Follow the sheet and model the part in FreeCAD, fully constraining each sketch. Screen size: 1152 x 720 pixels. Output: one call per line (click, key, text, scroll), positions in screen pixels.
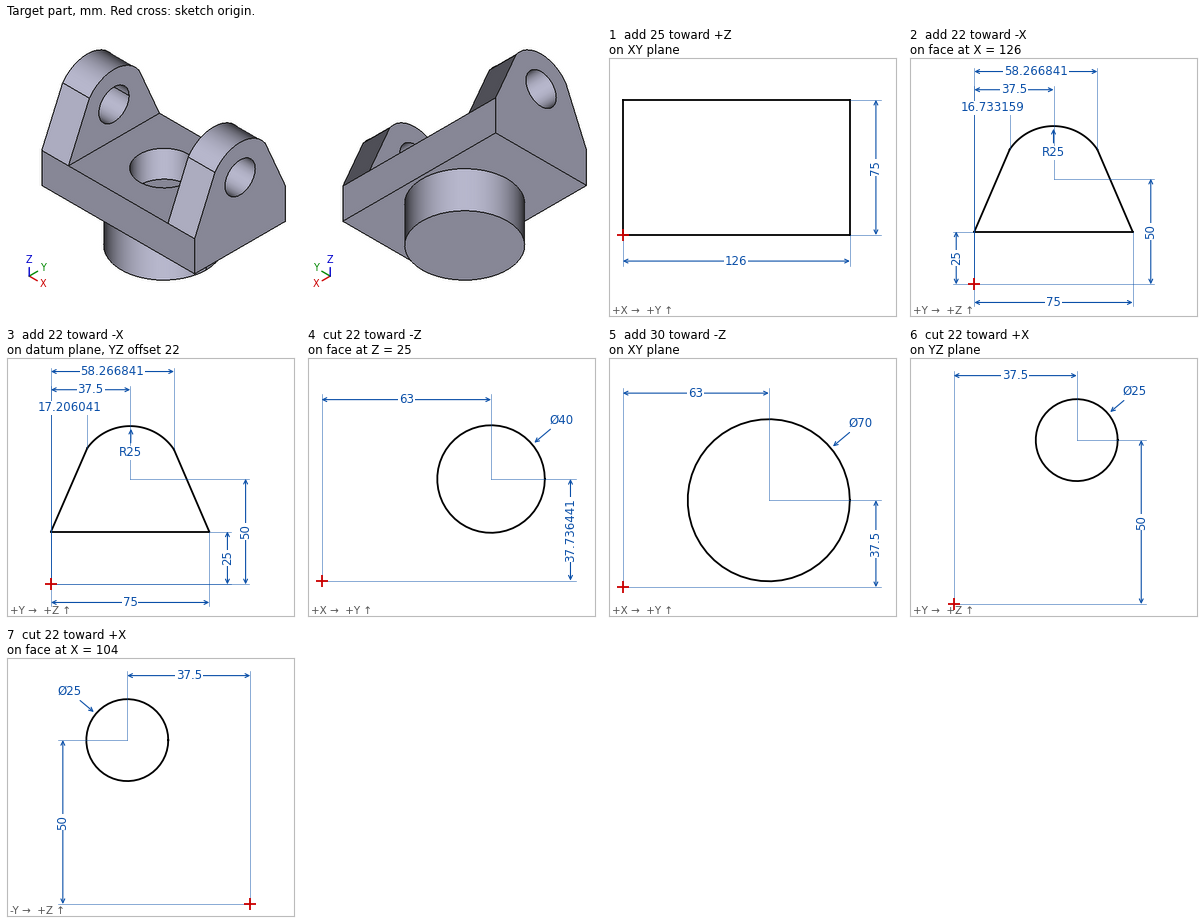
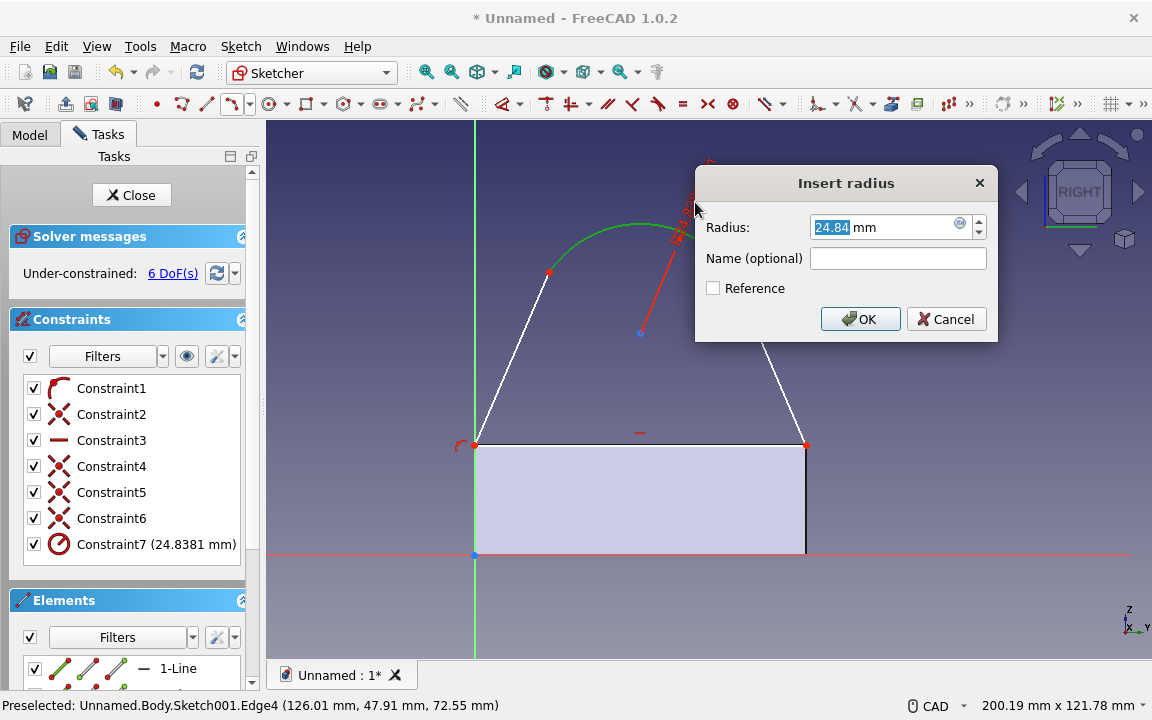
text(25)
key(Return)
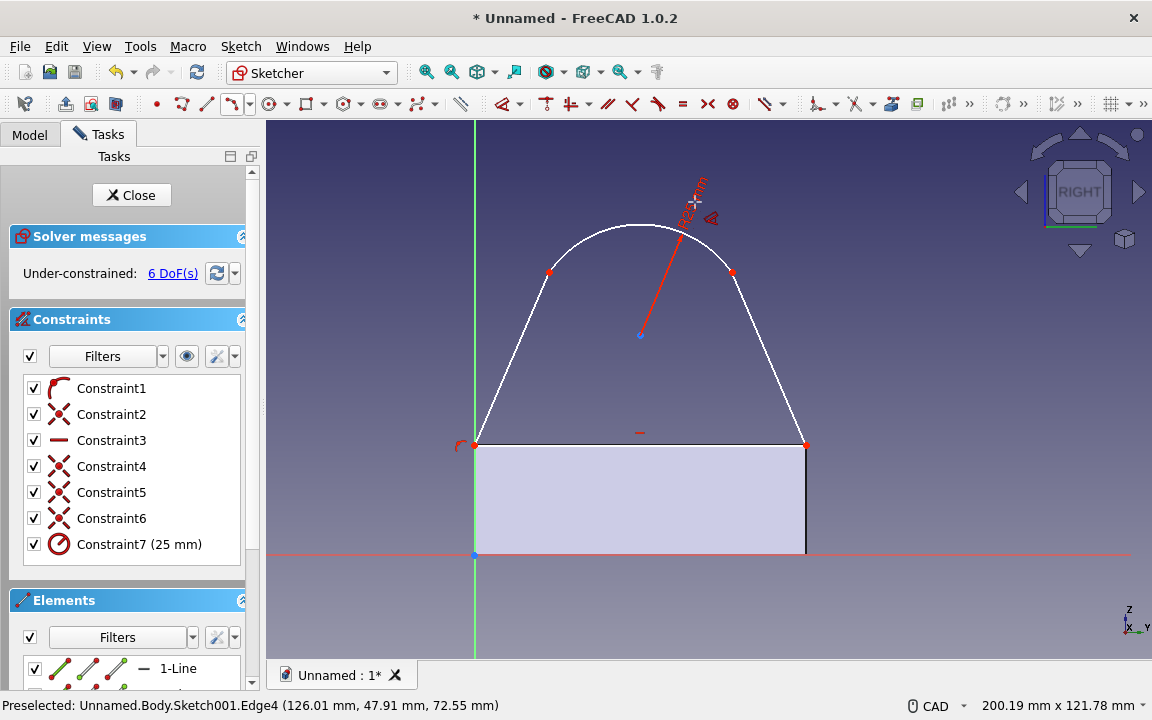
click(574, 446)
click(640, 480)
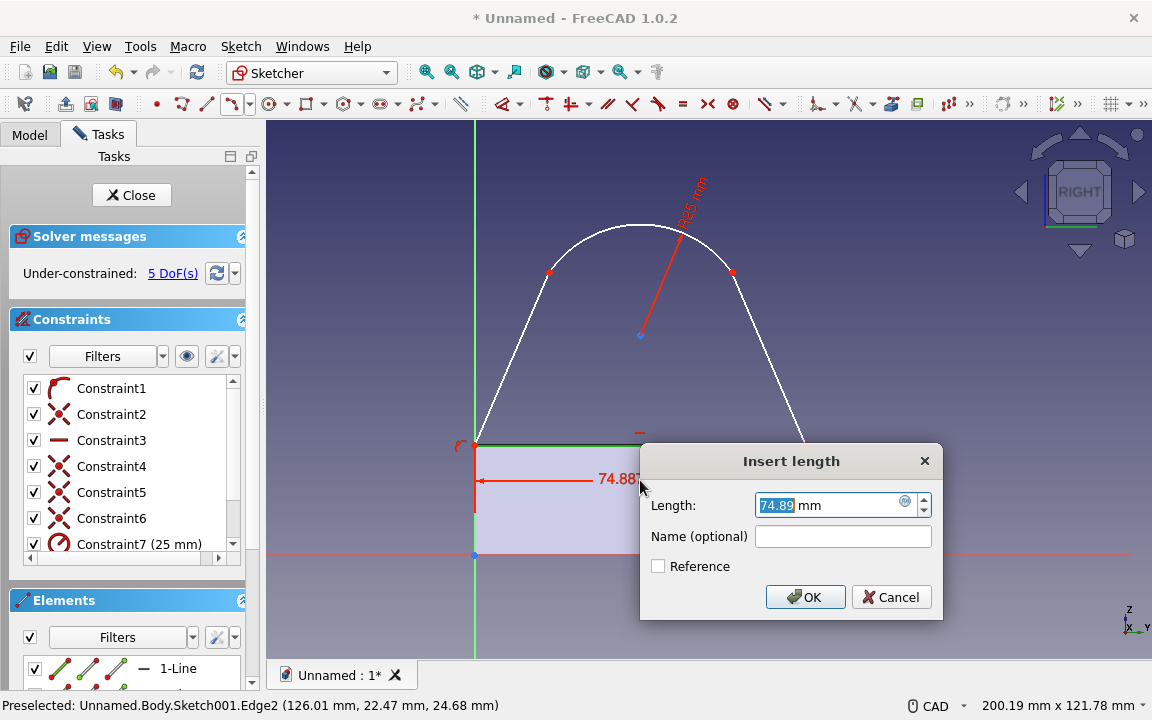
text(75)
key(Return)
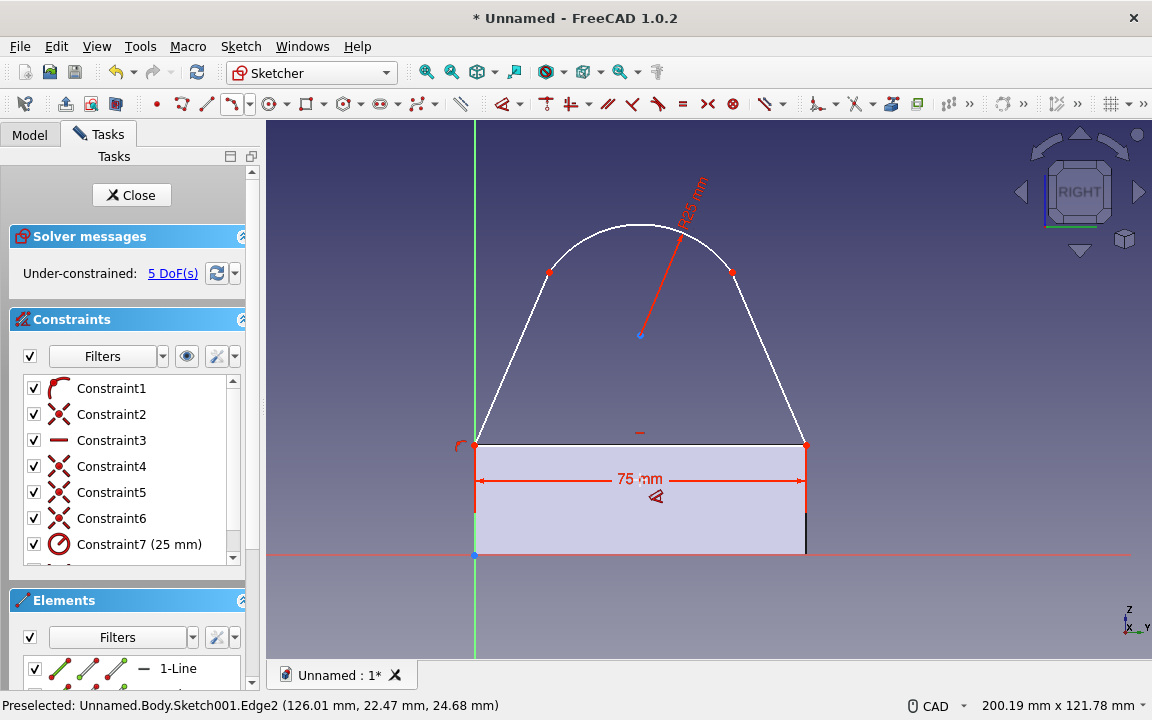
click(475, 446)
click(441, 501)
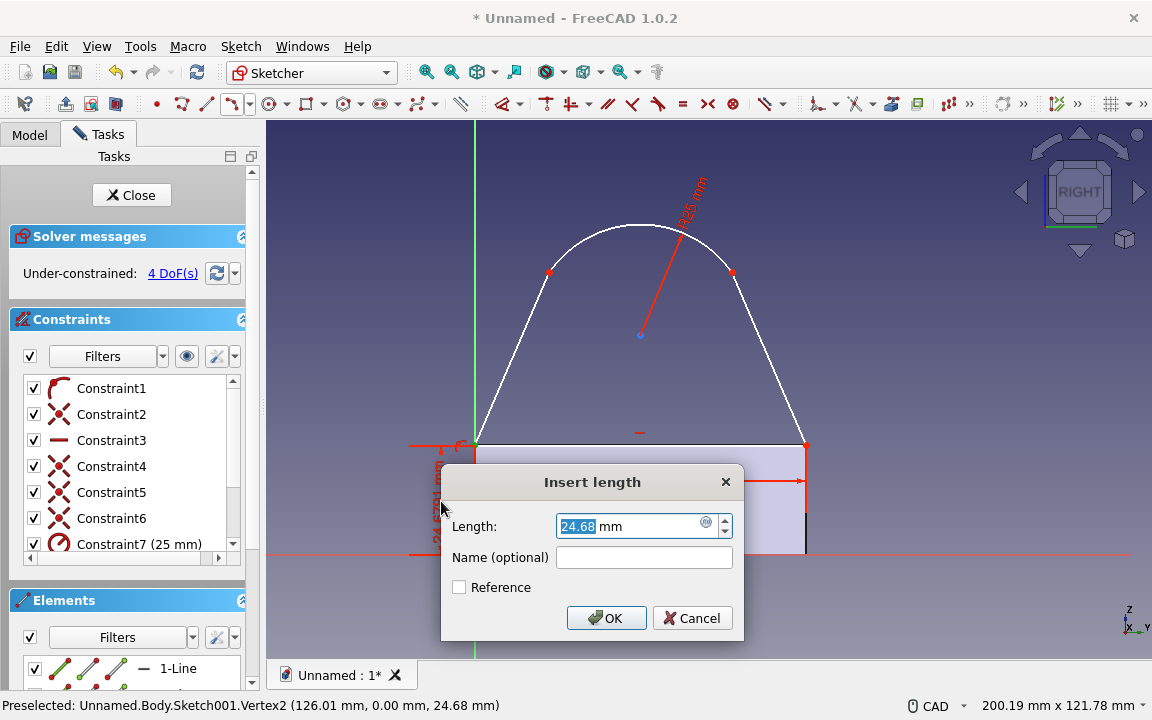
text(25)
key(Return)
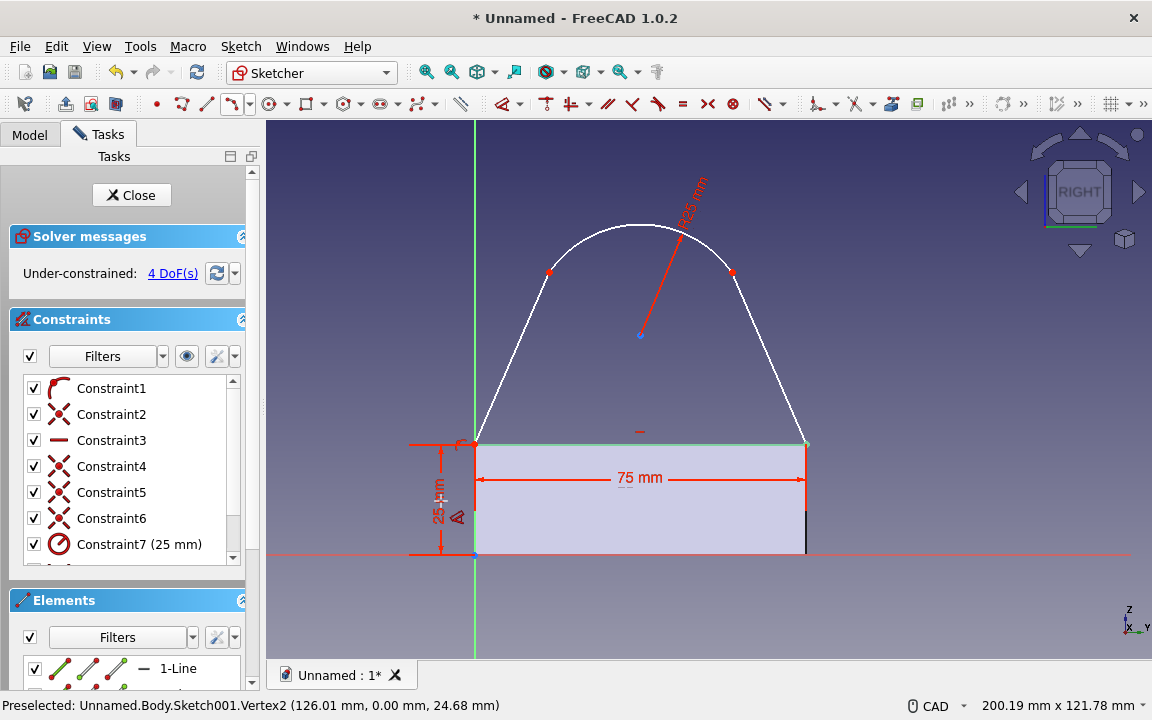
click(641, 335)
click(441, 445)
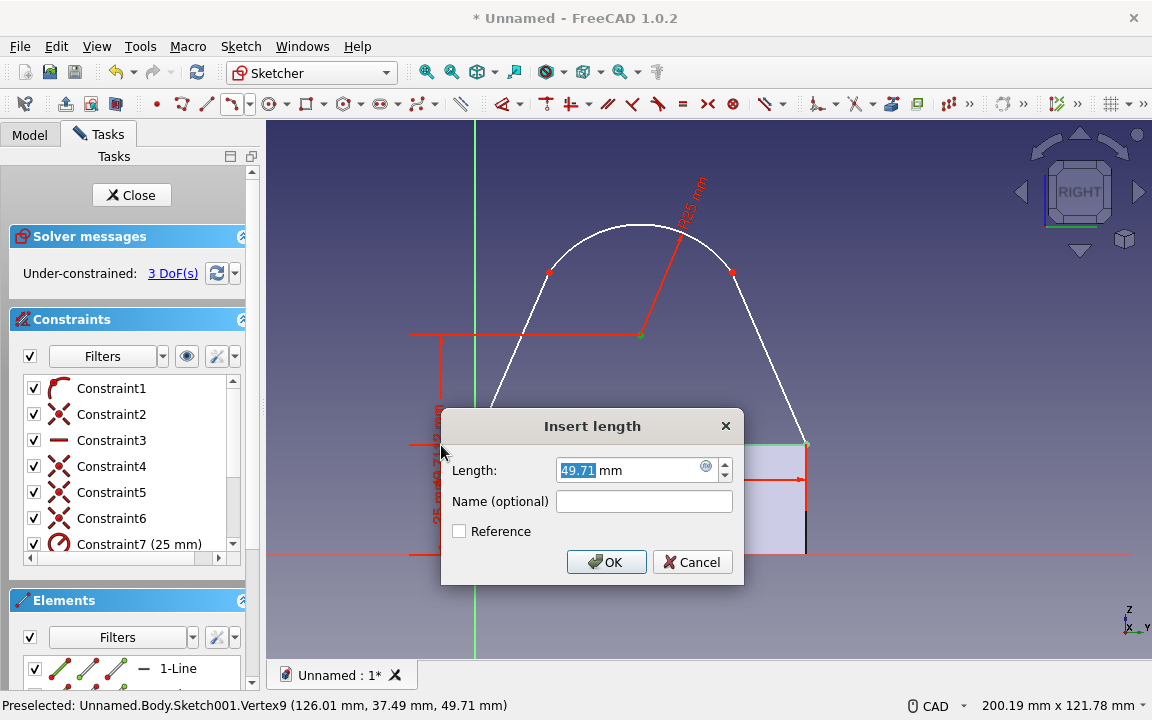
text(50)
key(Return)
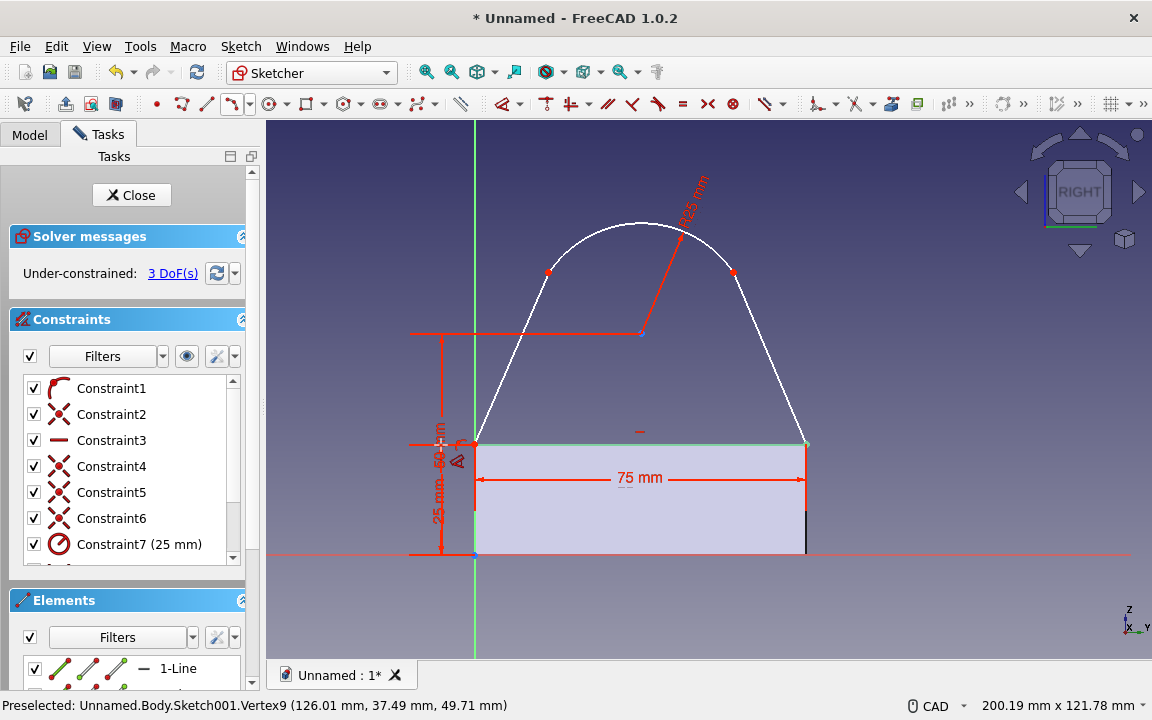
click(641, 334)
click(558, 589)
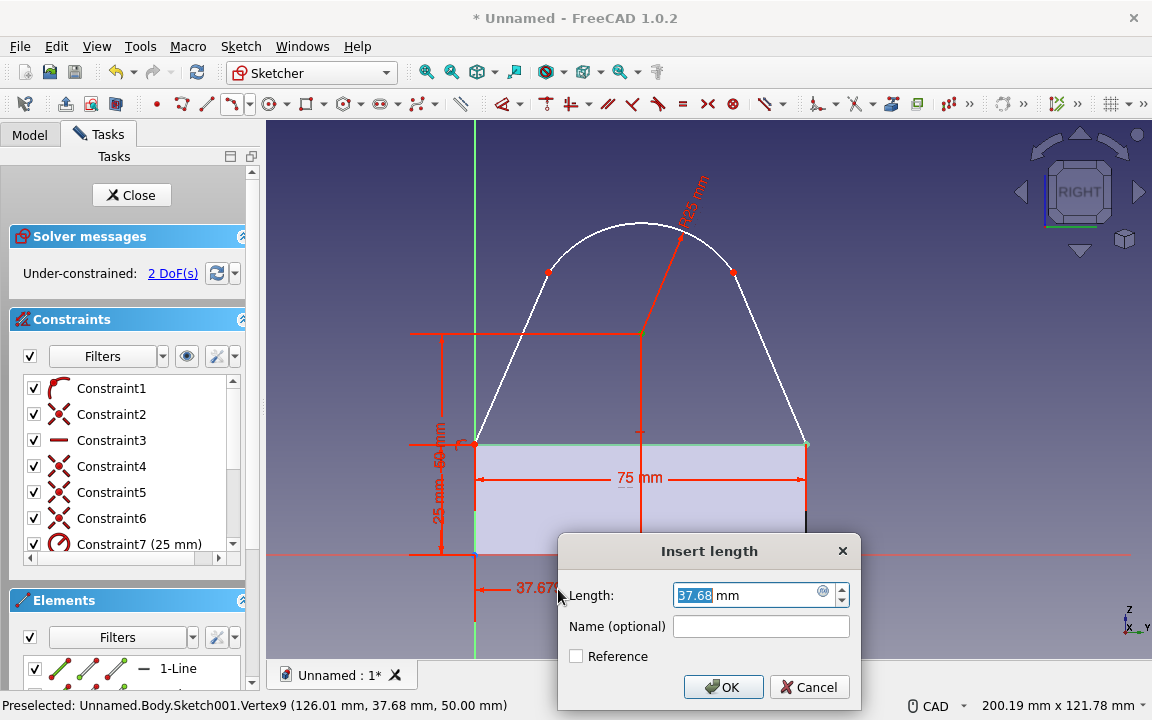
text(37.5)
key(Return)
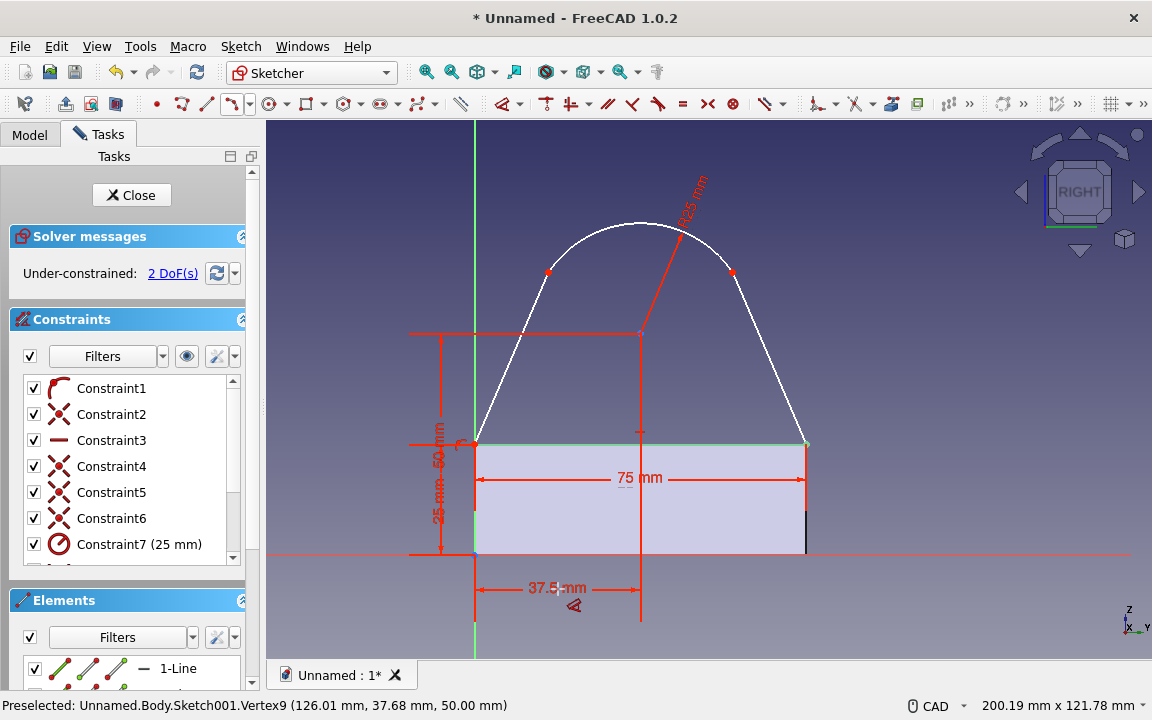
click(548, 273)
click(511, 239)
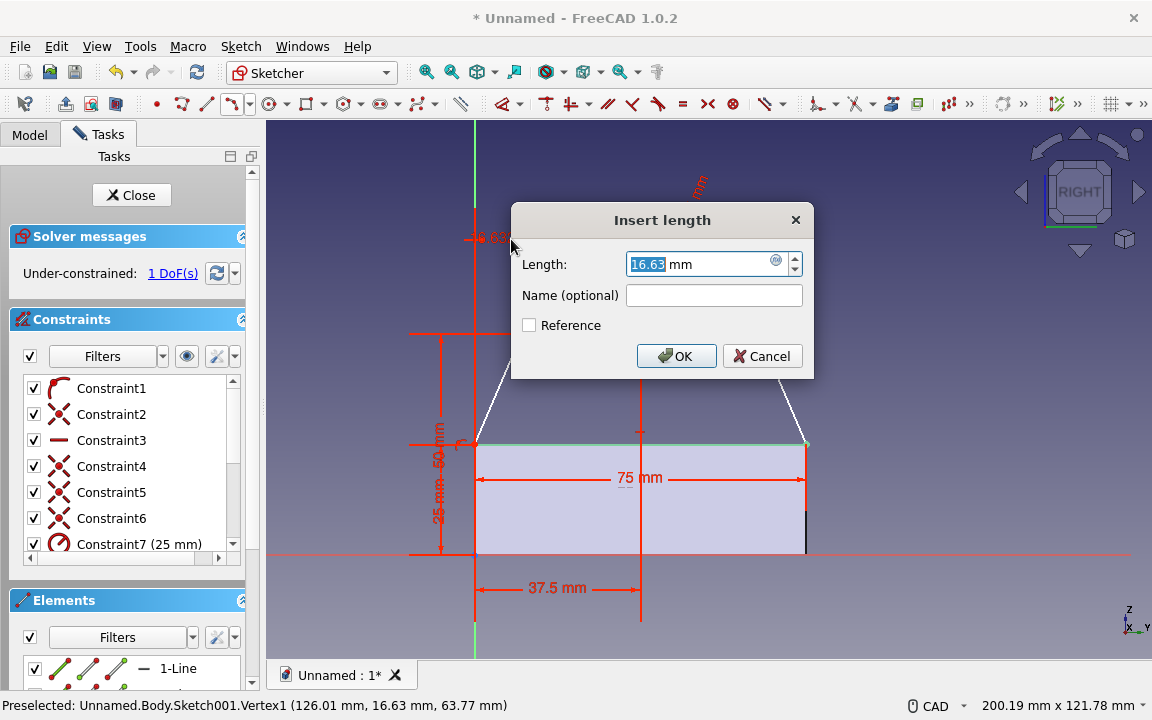
text(16.733159)
key(Return)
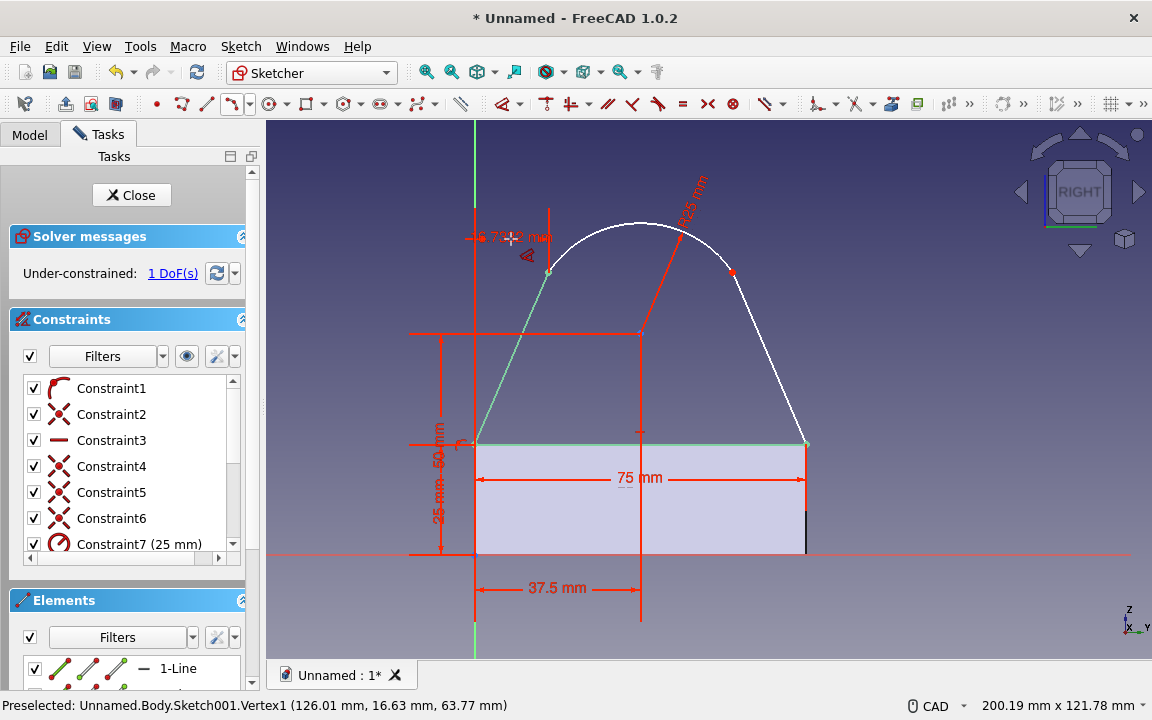
click(733, 273)
click(663, 589)